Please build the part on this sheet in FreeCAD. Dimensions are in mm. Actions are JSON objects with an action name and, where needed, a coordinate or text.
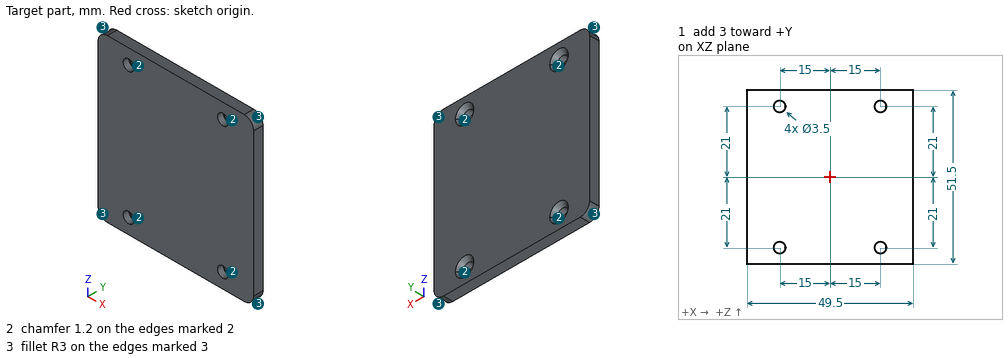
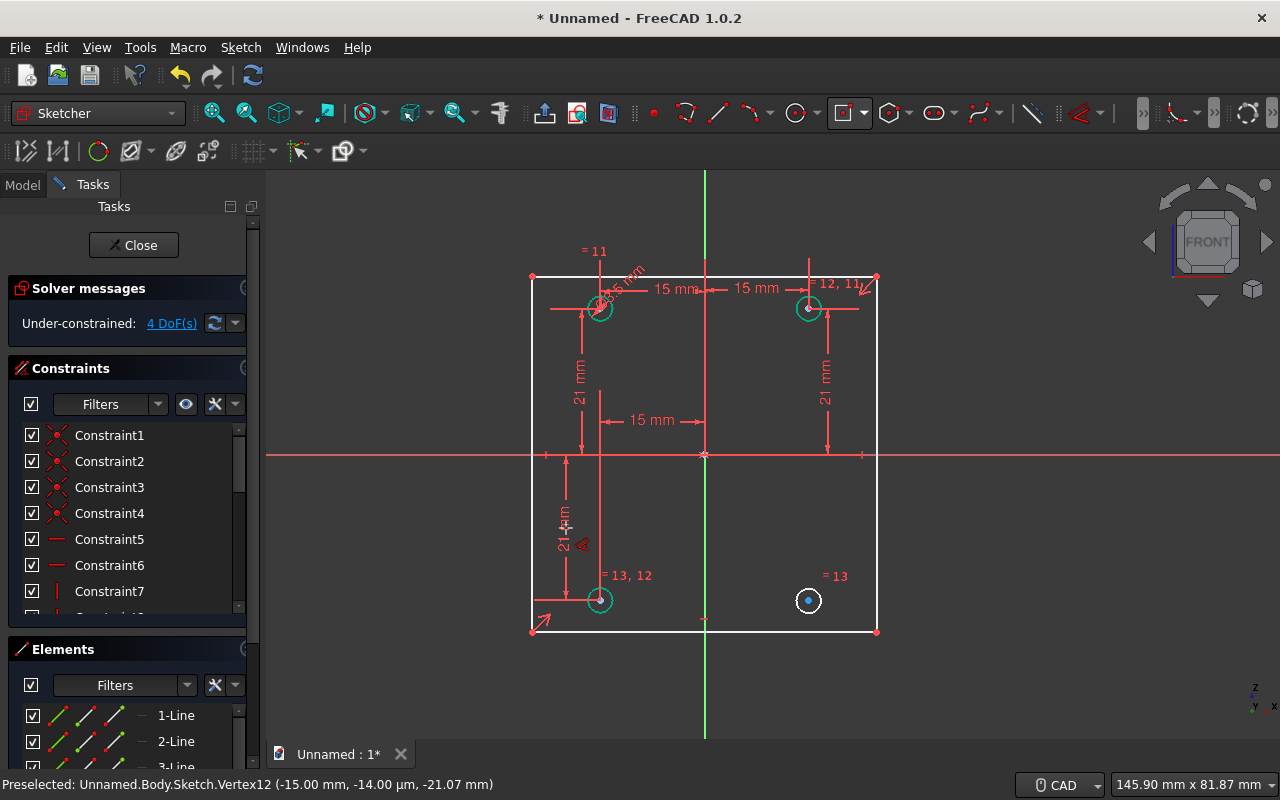
{"action": "left_click", "coordinate": [809, 601]}
{"action": "left_click", "coordinate": [757, 421]}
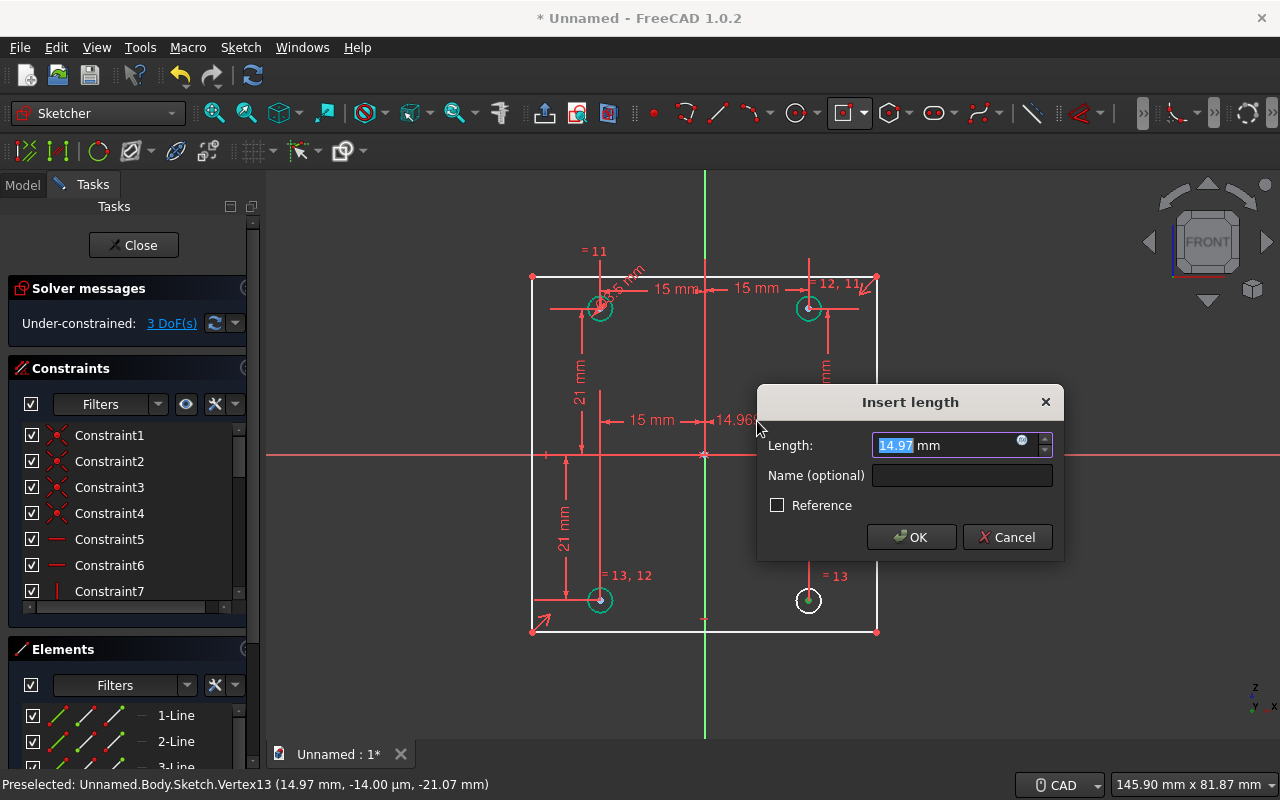
{"action": "type", "text": "15"}
{"action": "key", "text": "Return"}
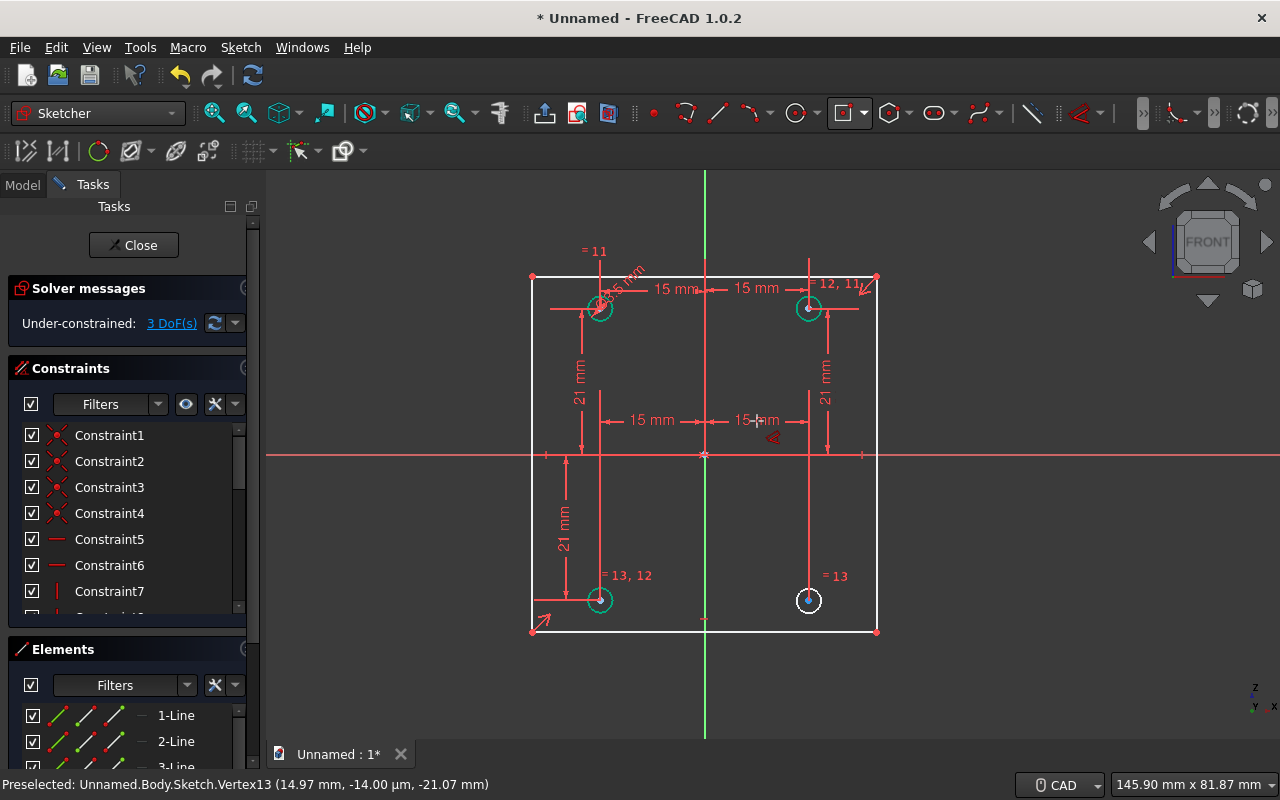
{"action": "left_click", "coordinate": [809, 601]}
{"action": "left_click", "coordinate": [843, 528]}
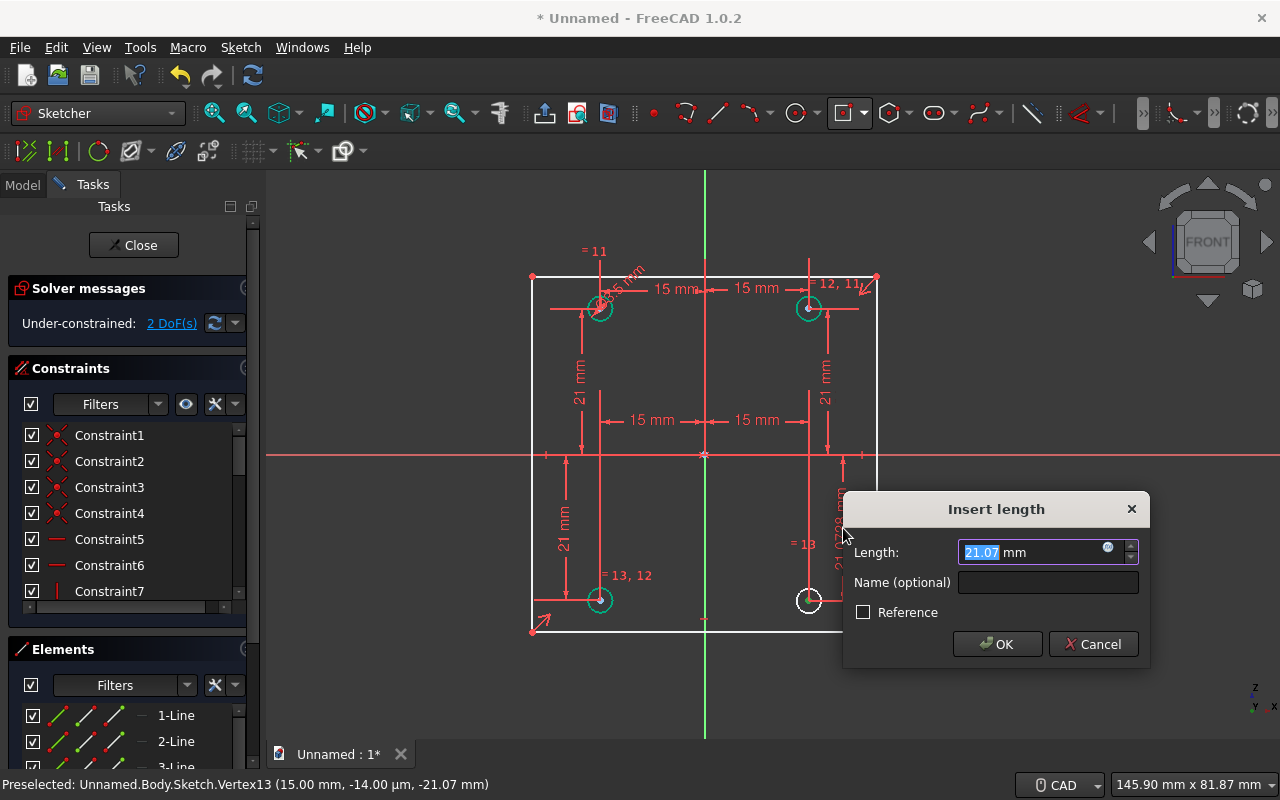
{"action": "type", "text": "21"}
{"action": "key", "text": "Return"}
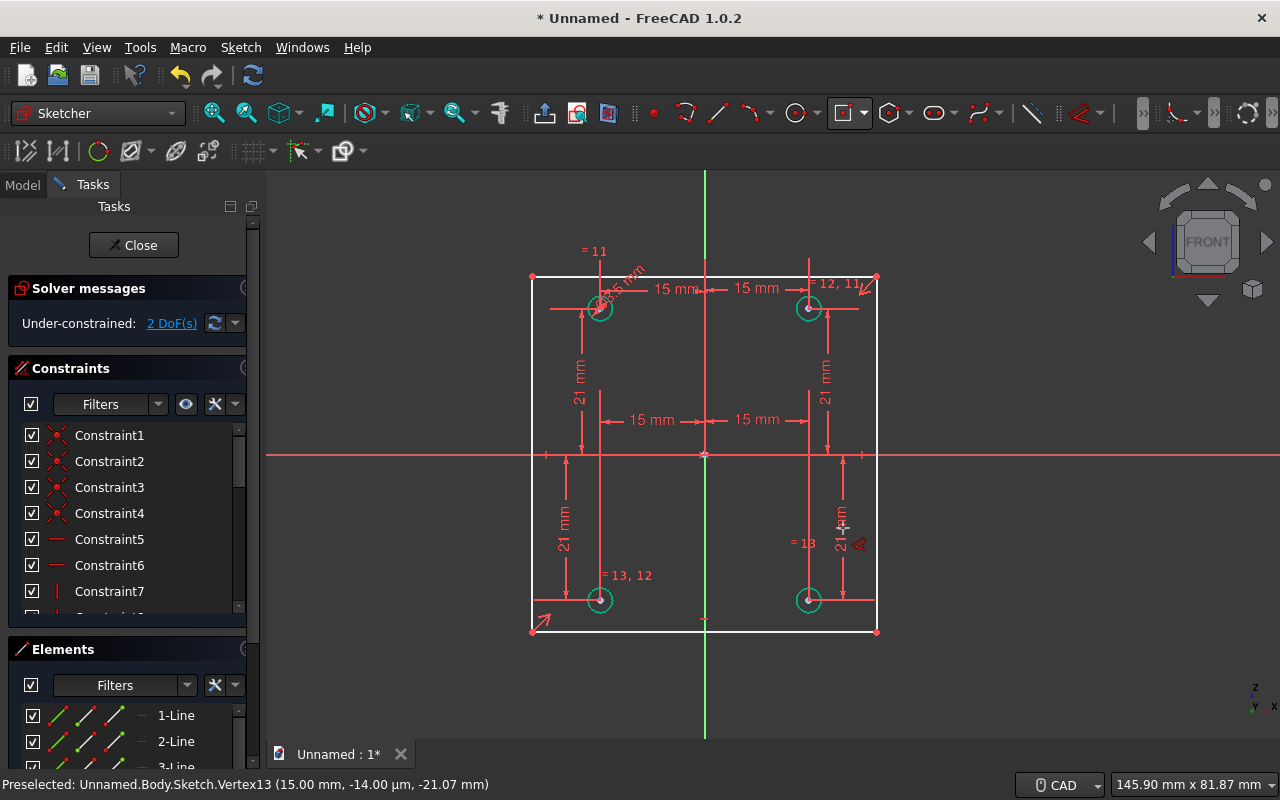
{"action": "left_click", "coordinate": [636, 632]}
{"action": "left_click", "coordinate": [625, 666]}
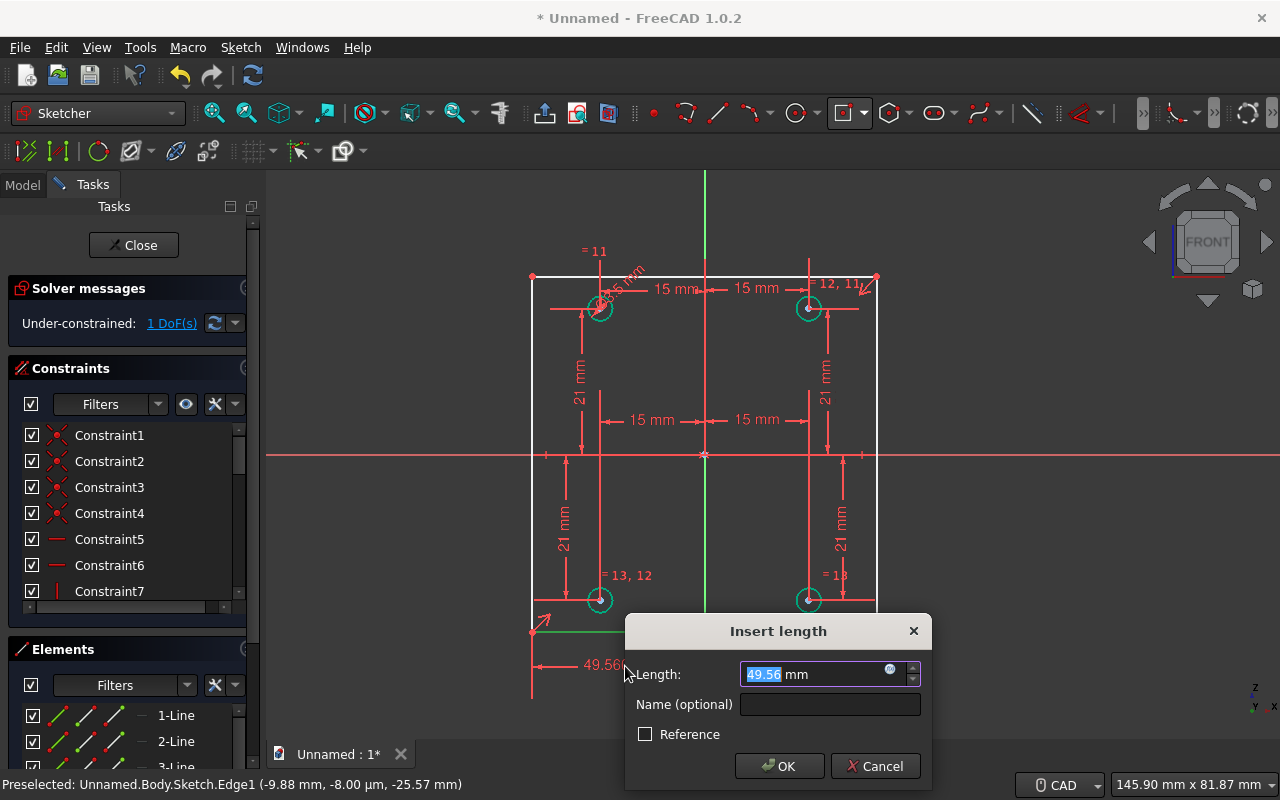
{"action": "type", "text": "49.5"}
{"action": "key", "text": "Return"}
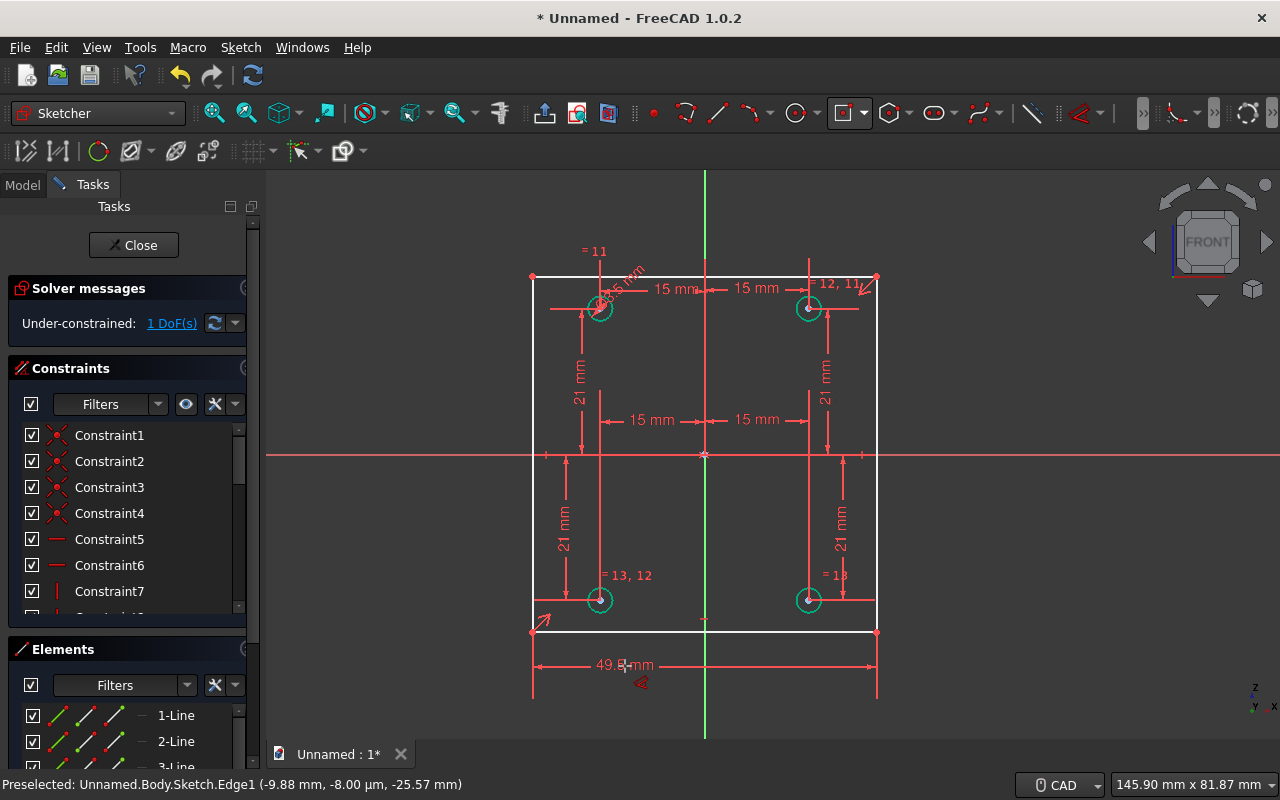
{"action": "left_click", "coordinate": [877, 526]}
{"action": "left_click", "coordinate": [911, 373]}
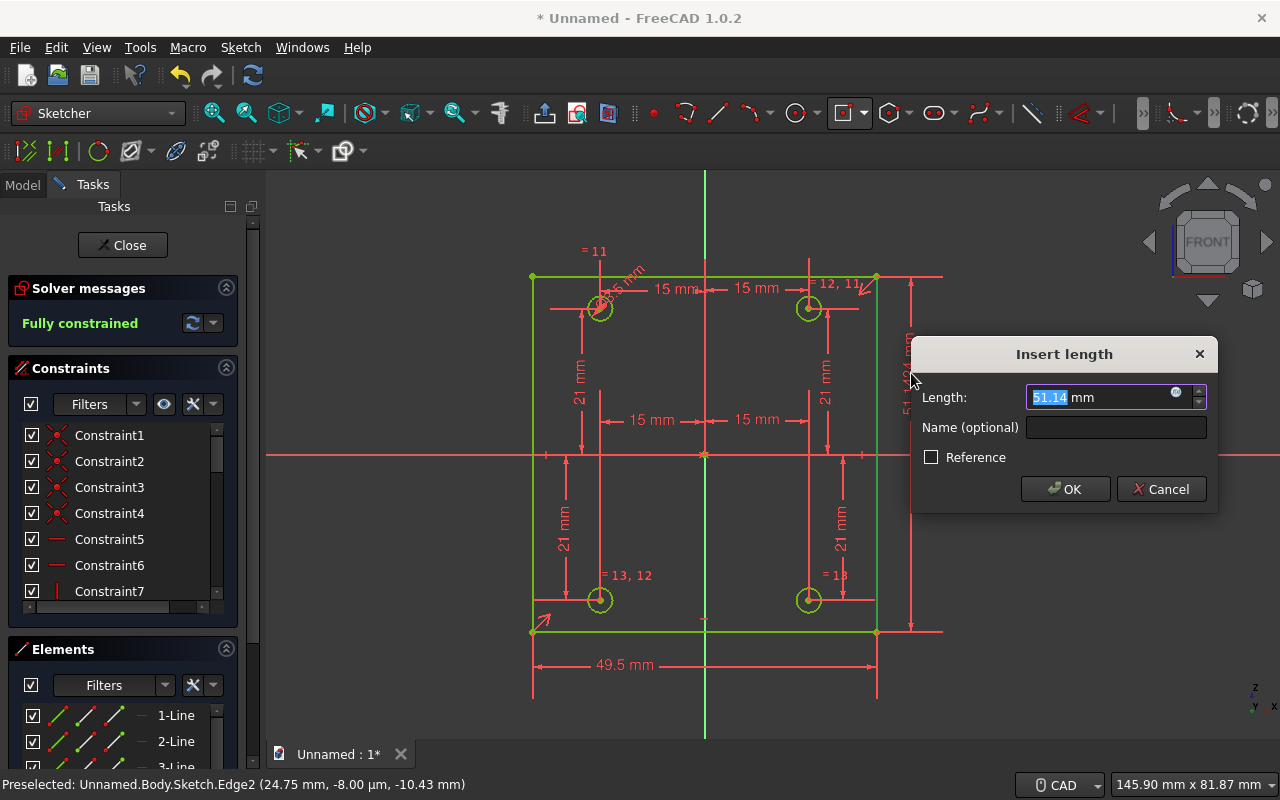
{"action": "type", "text": "51.5"}
{"action": "key", "text": "Return"}
{"action": "key", "text": "Escape"}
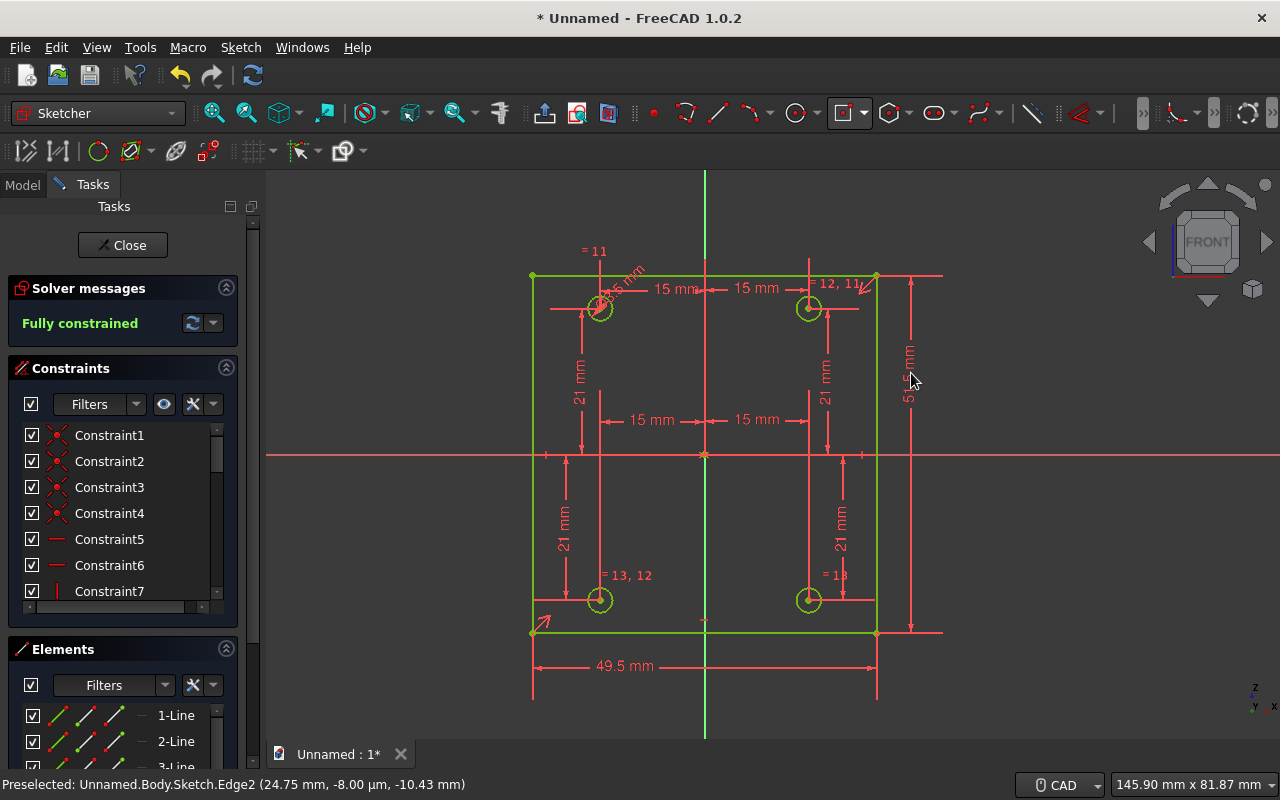
{"action": "left_click", "coordinate": [123, 245]}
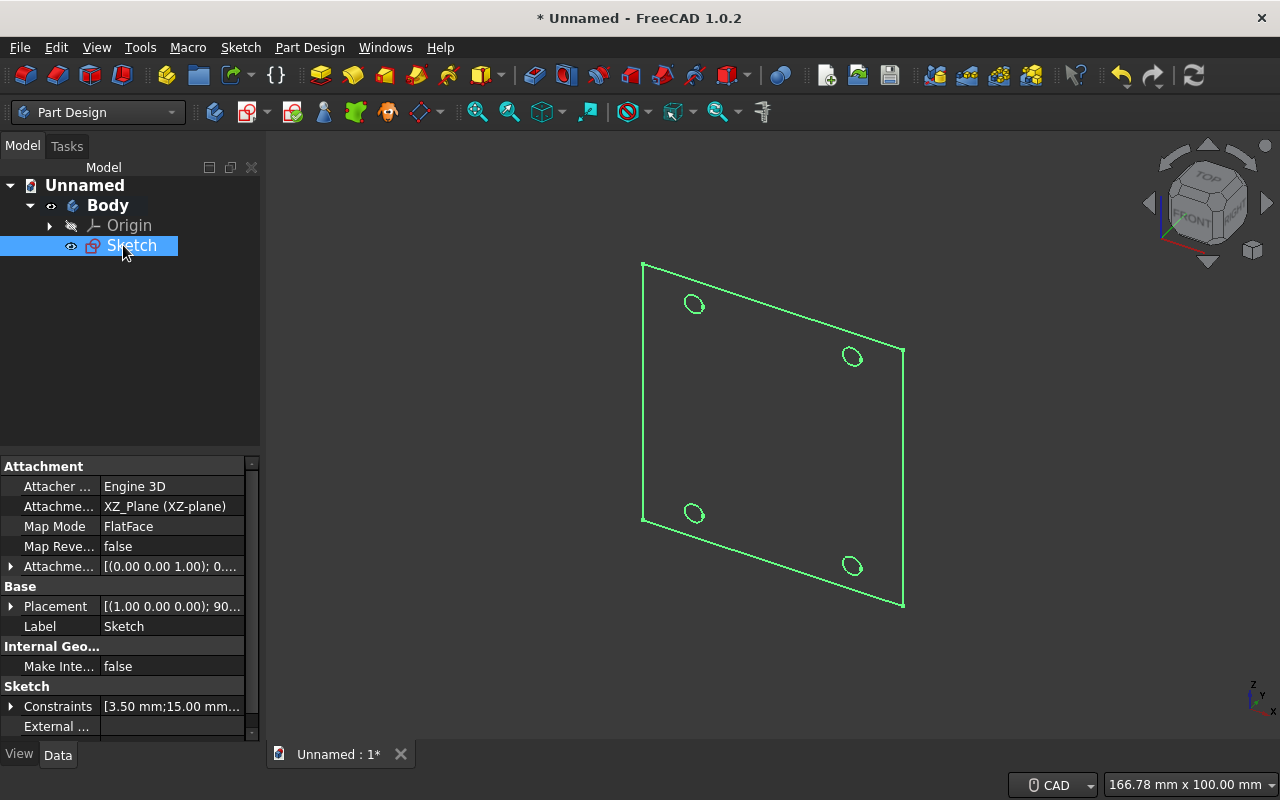
{"action": "left_click", "coordinate": [322, 76]}